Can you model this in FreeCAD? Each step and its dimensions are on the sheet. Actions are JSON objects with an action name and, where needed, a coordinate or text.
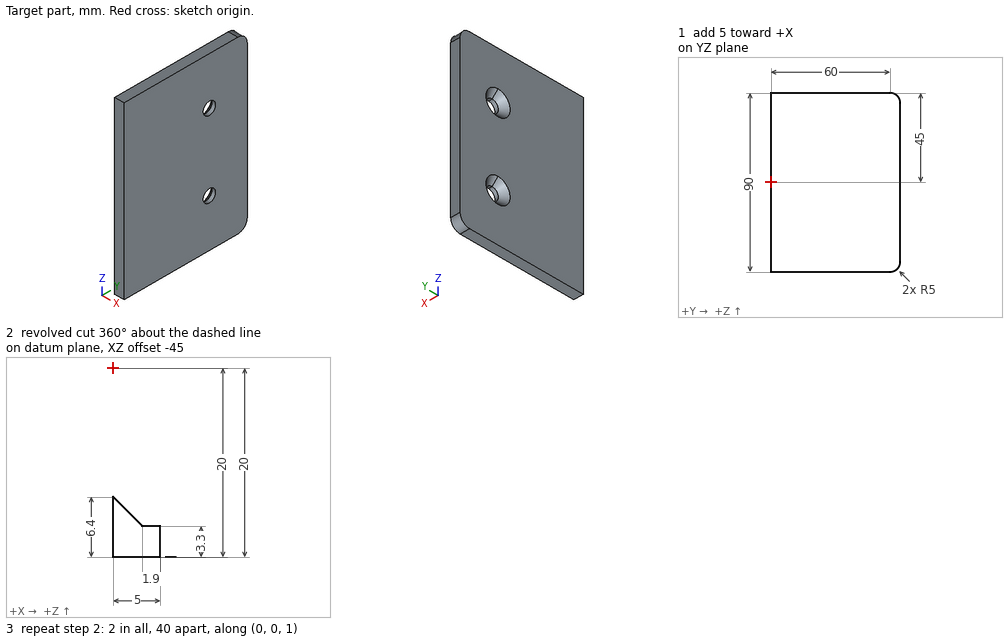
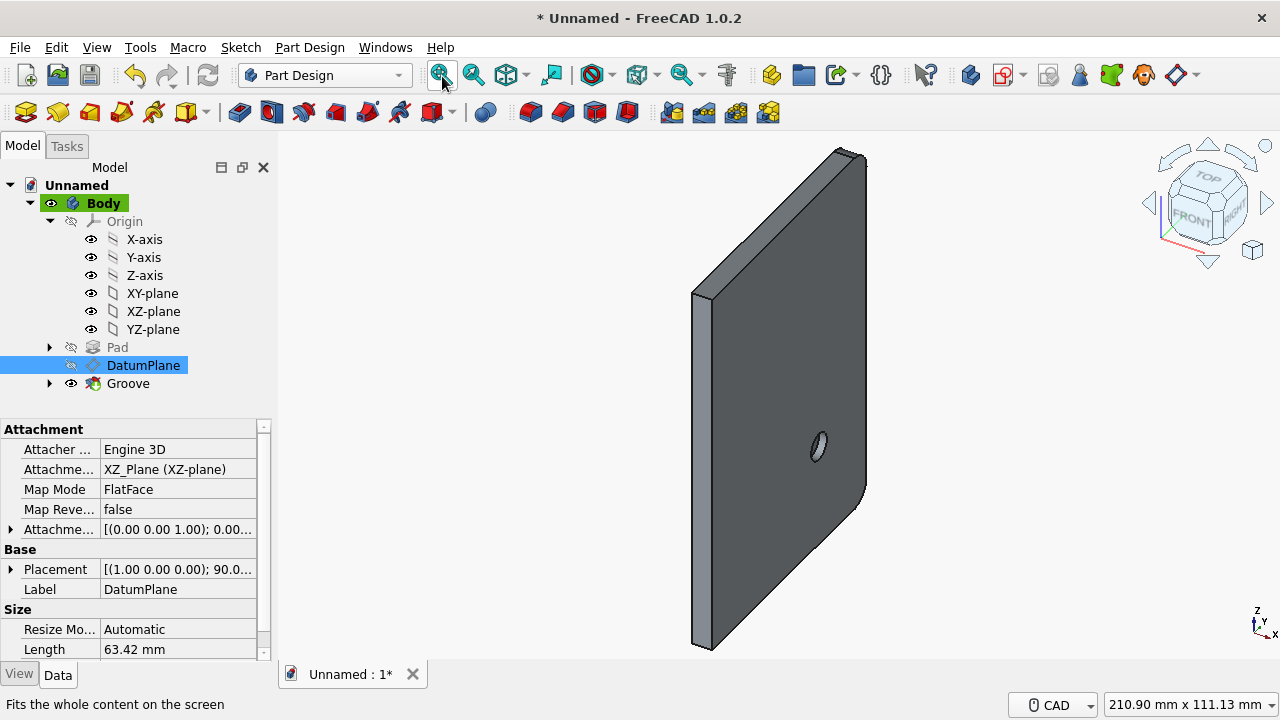
{"action": "left_click", "coordinate": [116, 383]}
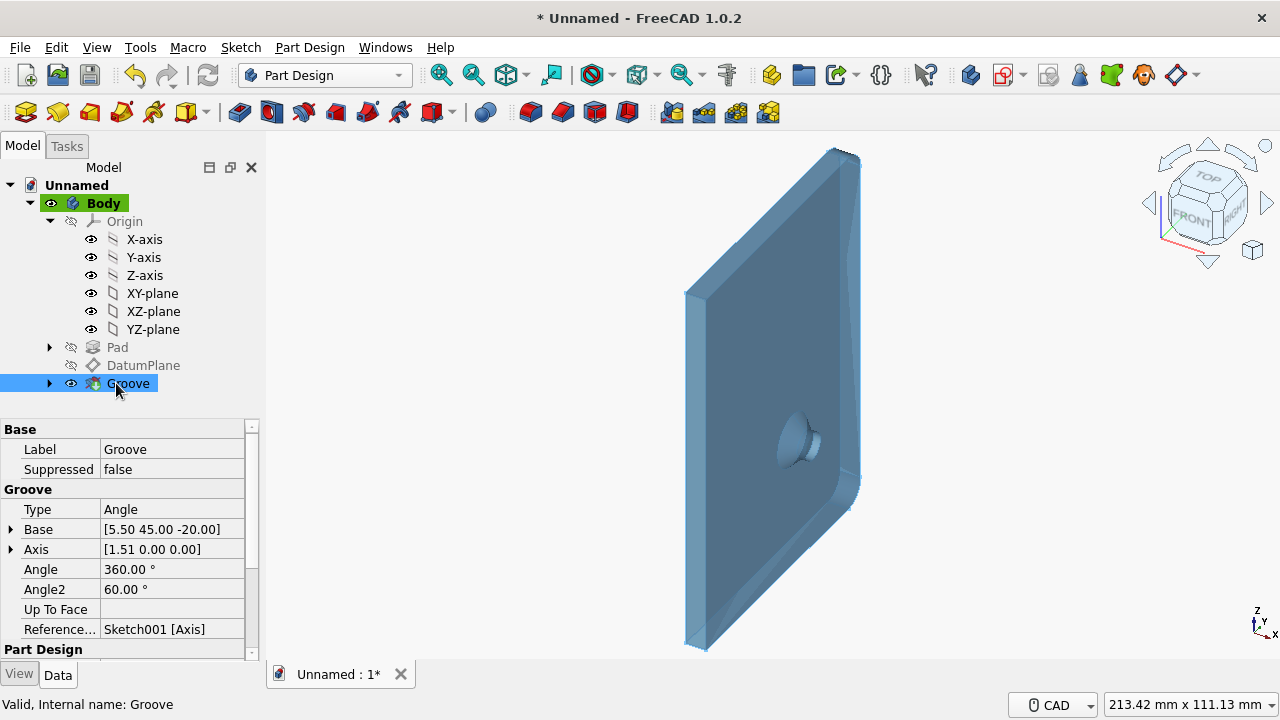
{"action": "left_click", "coordinate": [704, 112]}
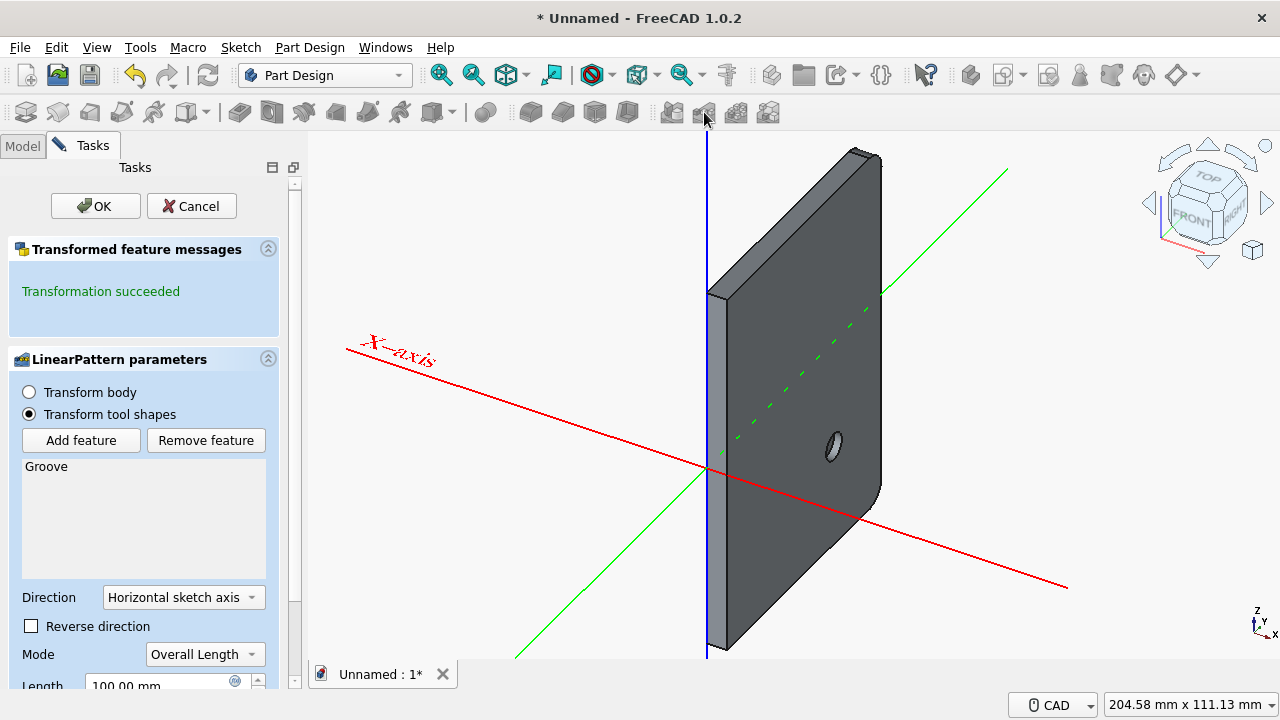
{"action": "left_click", "coordinate": [184, 598]}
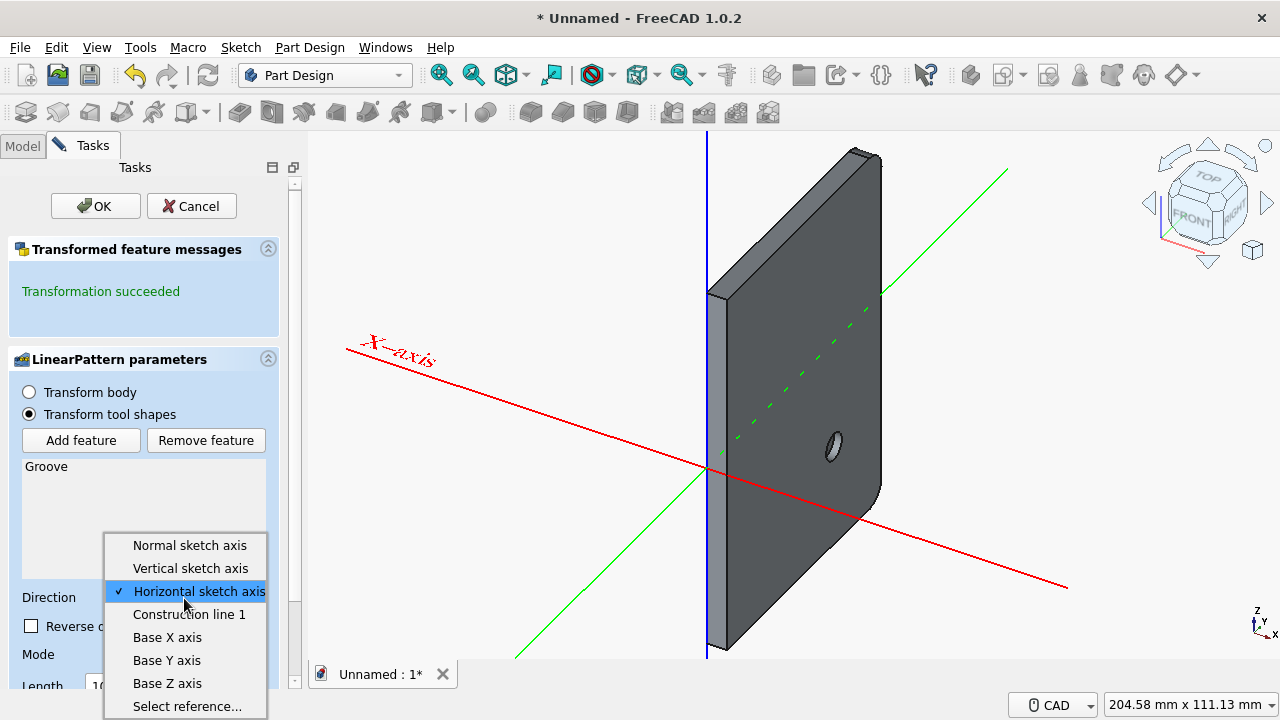
{"action": "left_click", "coordinate": [184, 684]}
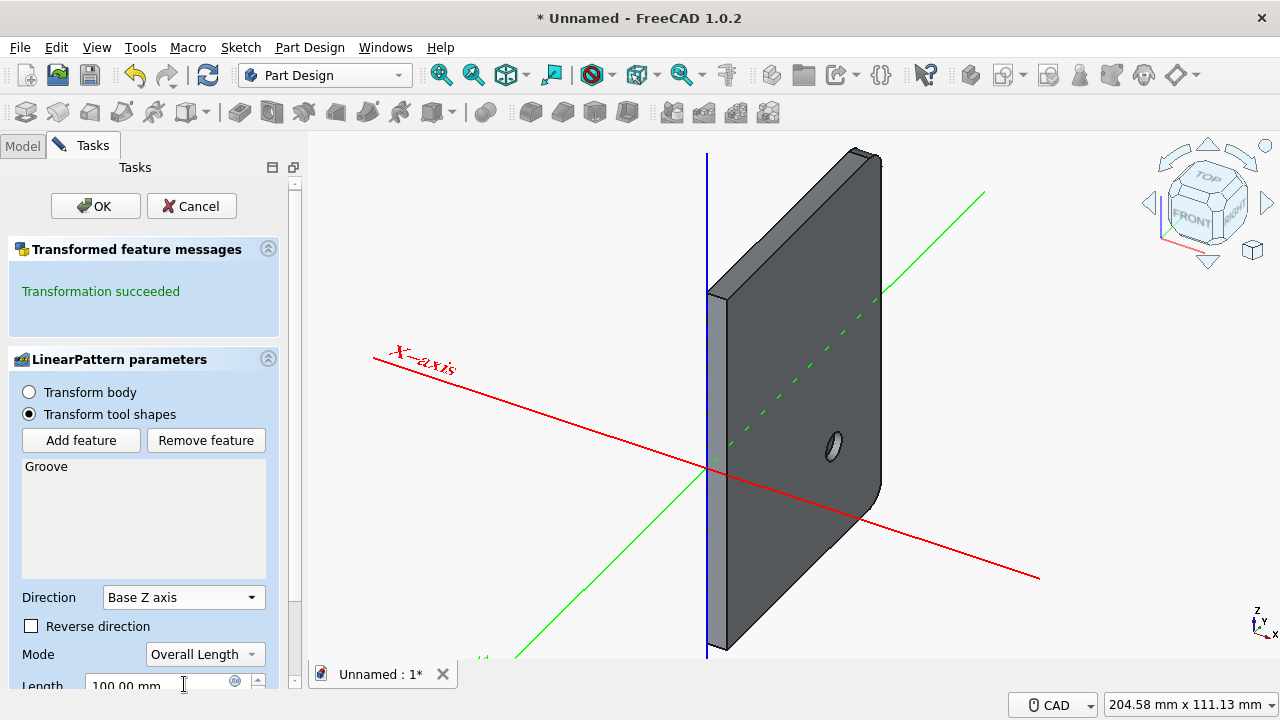
{"action": "left_click", "coordinate": [206, 654]}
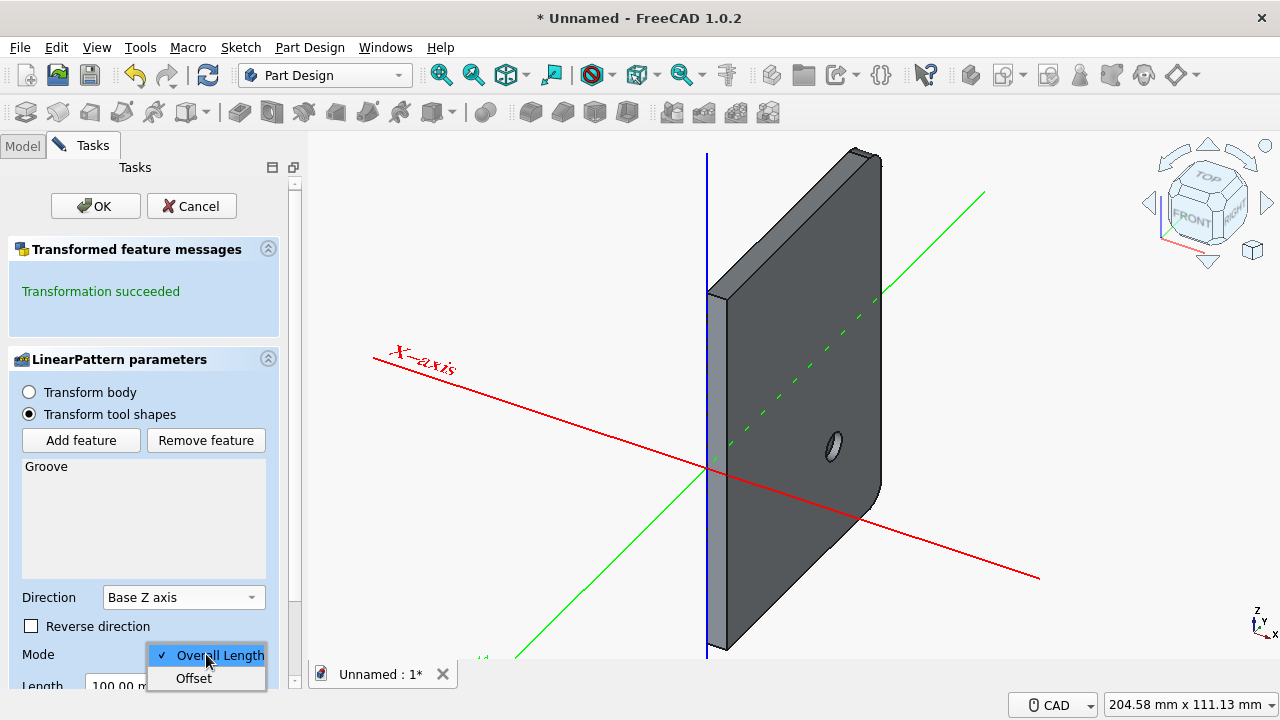
{"action": "left_click", "coordinate": [206, 678]}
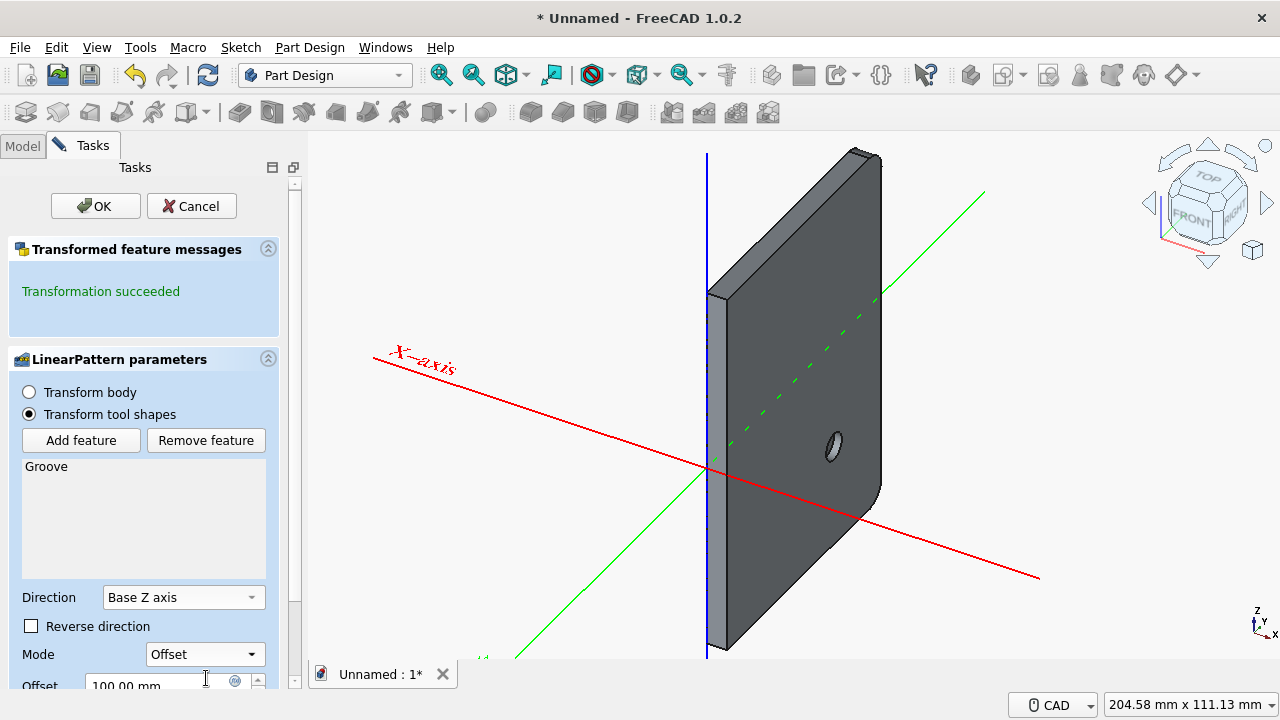
{"action": "scroll", "coordinate": [295, 432], "scroll_direction": "down", "scroll_amount": 2}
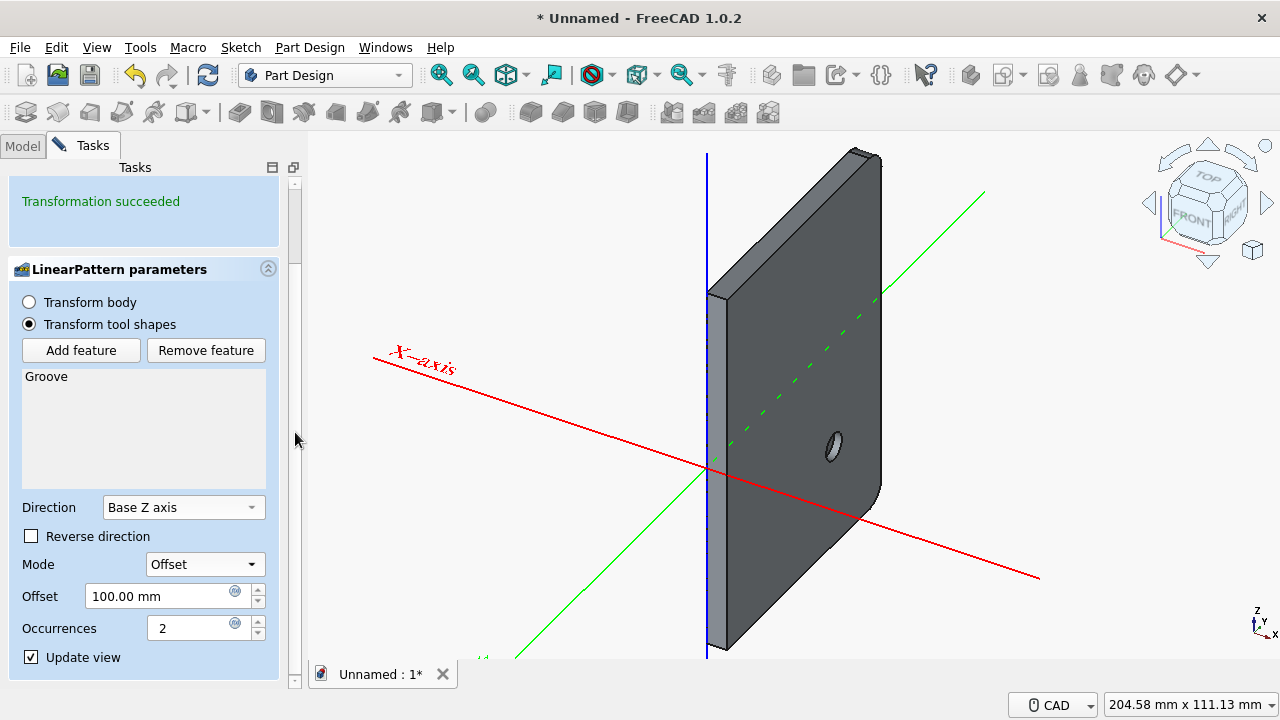
{"action": "triple_click", "coordinate": [168, 596]}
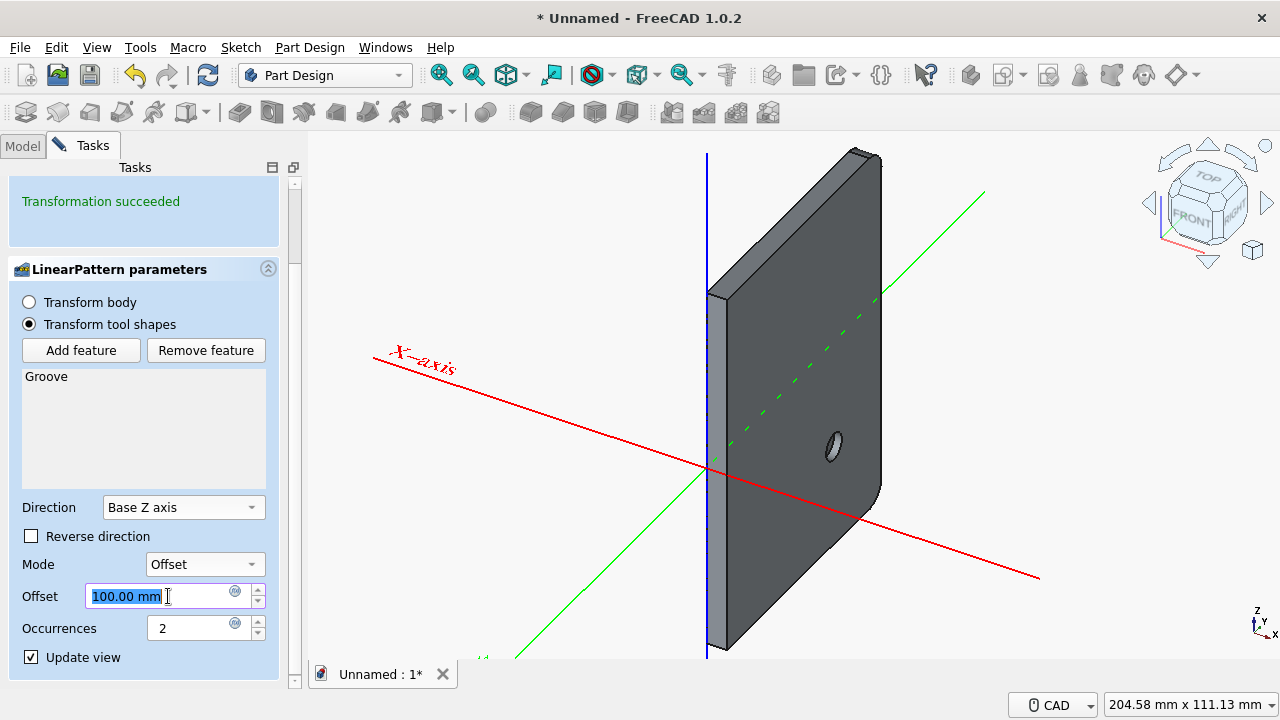
{"action": "type", "text": "40"}
{"action": "key", "text": "Tab"}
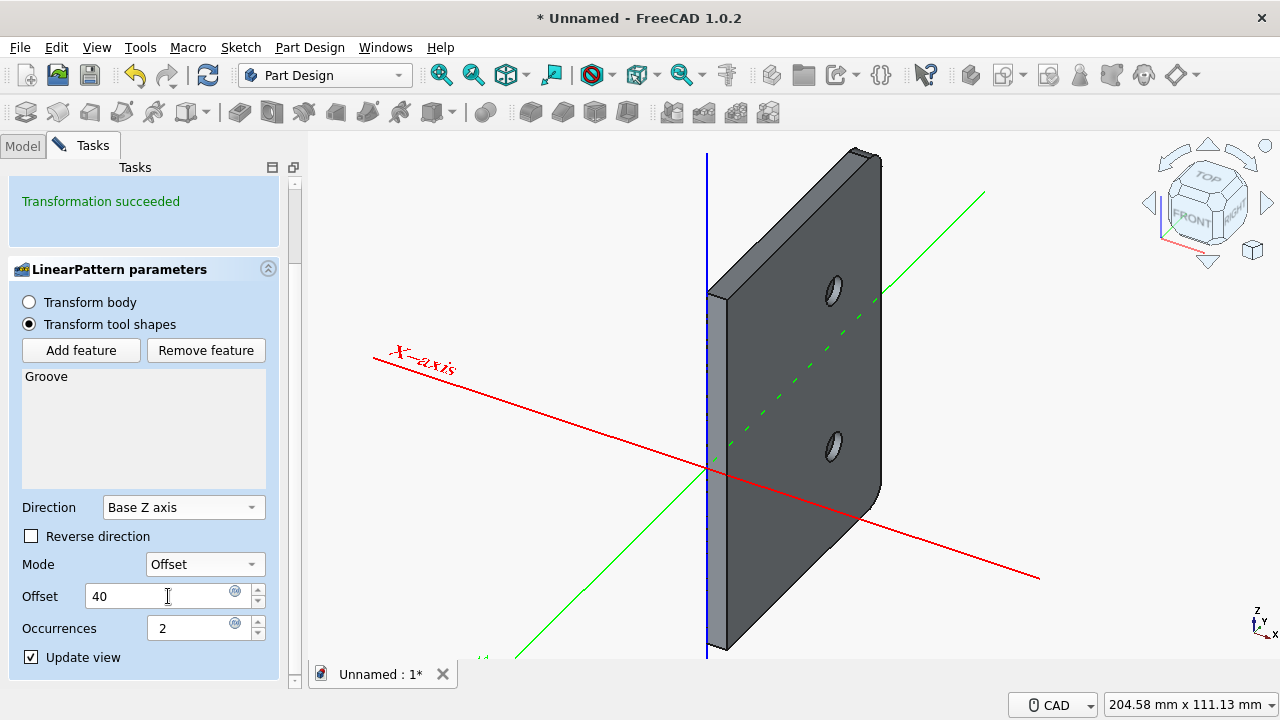
{"action": "triple_click", "coordinate": [198, 628]}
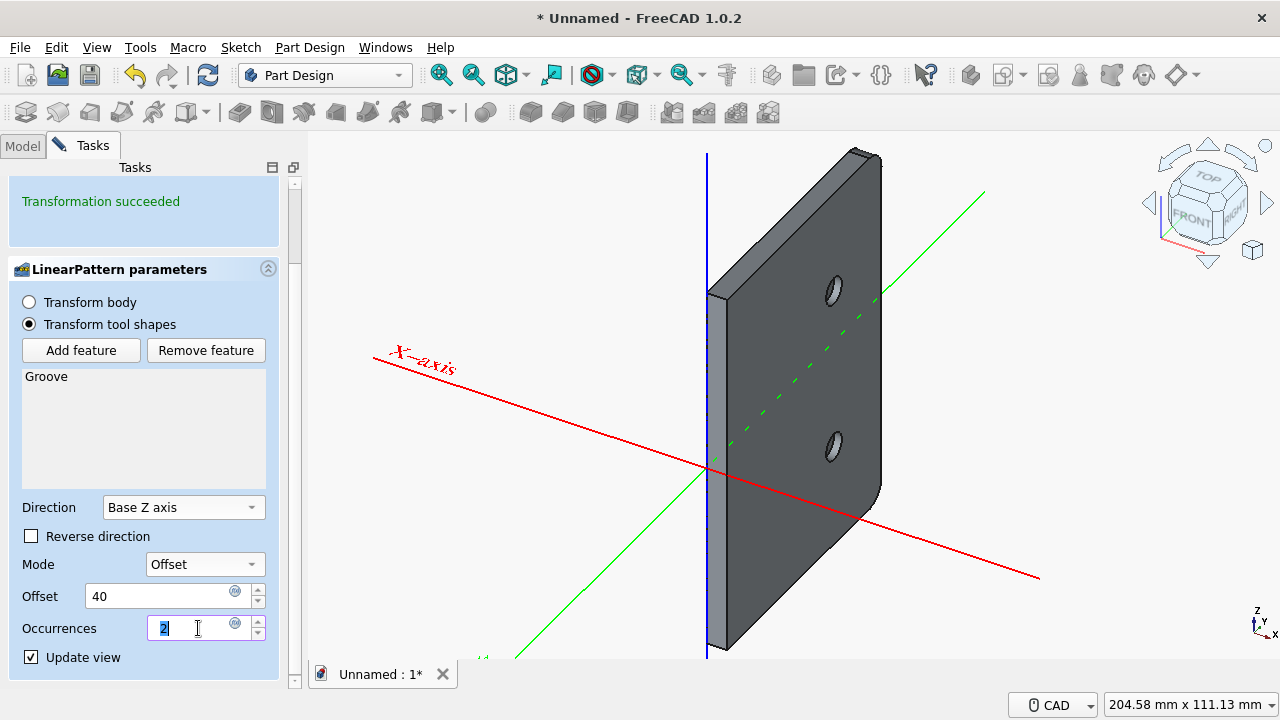
{"action": "type", "text": "2"}
{"action": "key", "text": "Tab"}